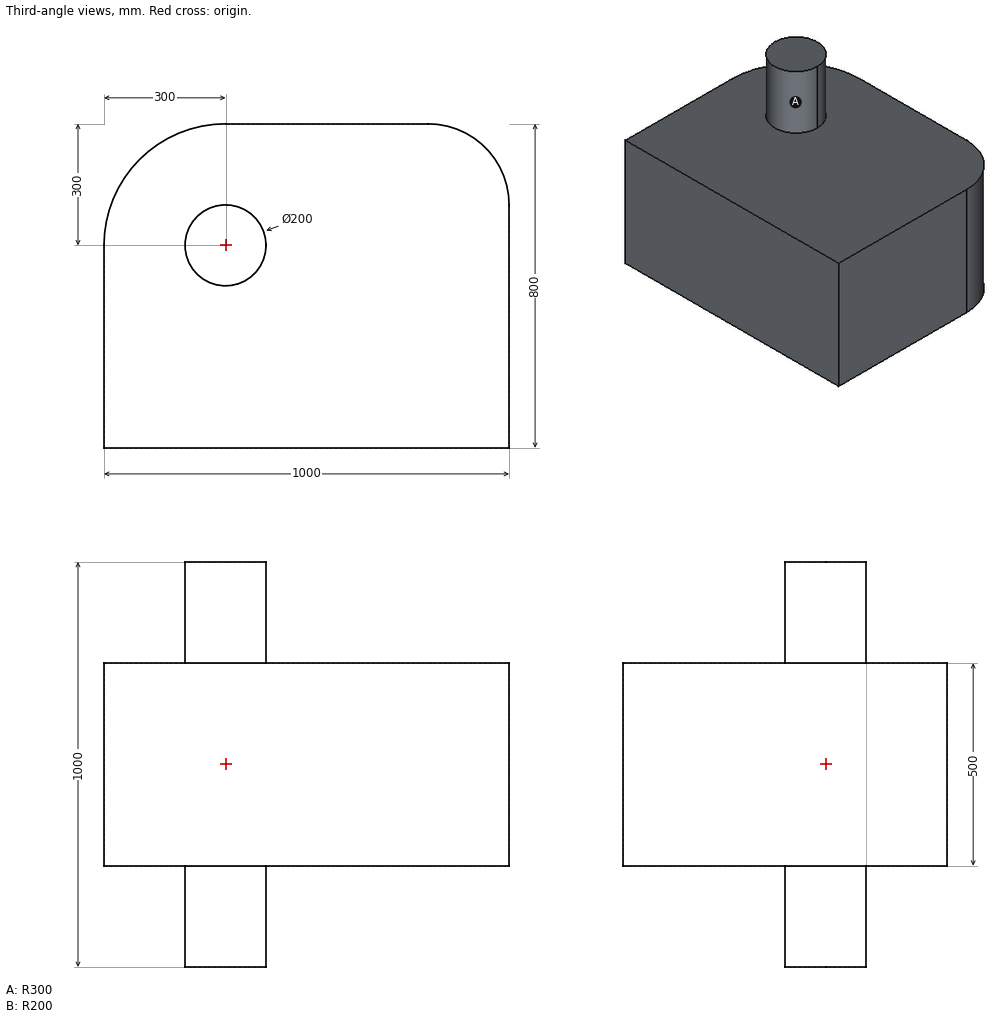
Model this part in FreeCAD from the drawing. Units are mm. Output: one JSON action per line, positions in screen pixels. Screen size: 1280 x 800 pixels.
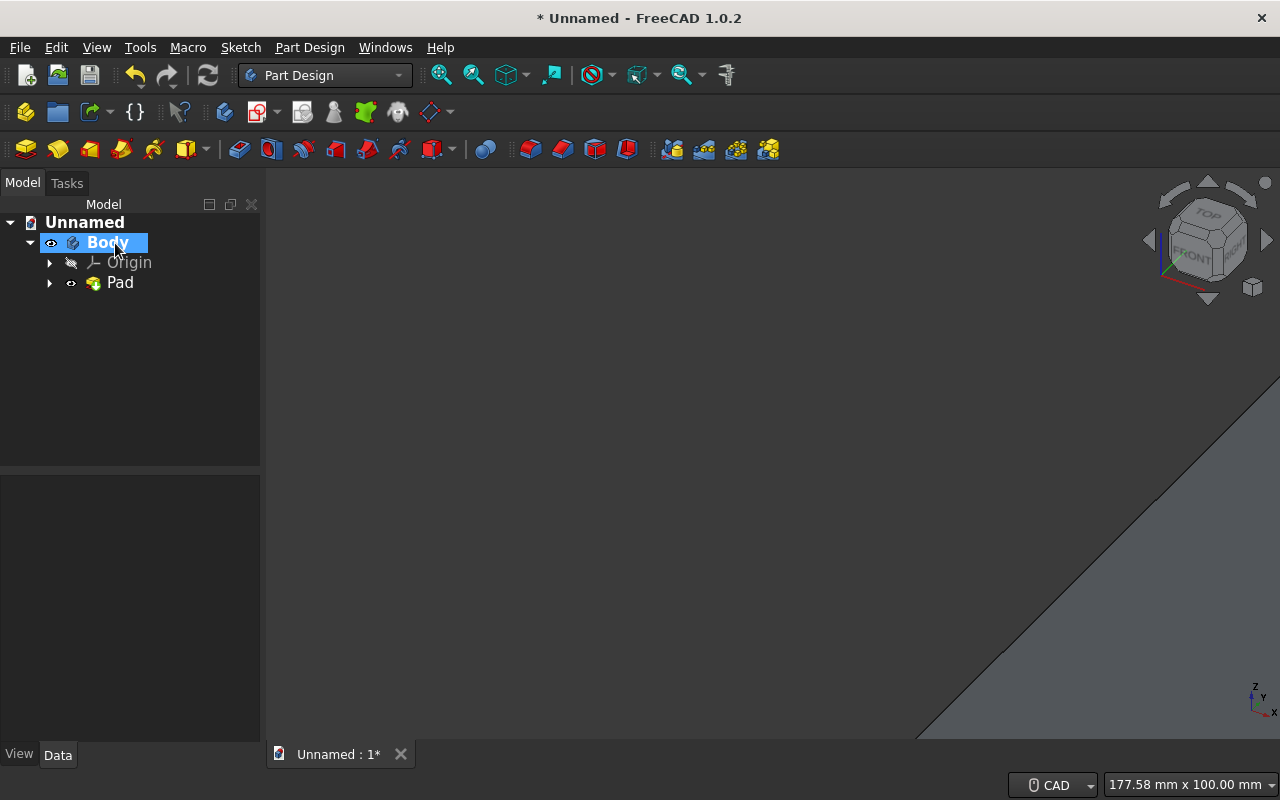
{"action": "left_click", "coordinate": [442, 76]}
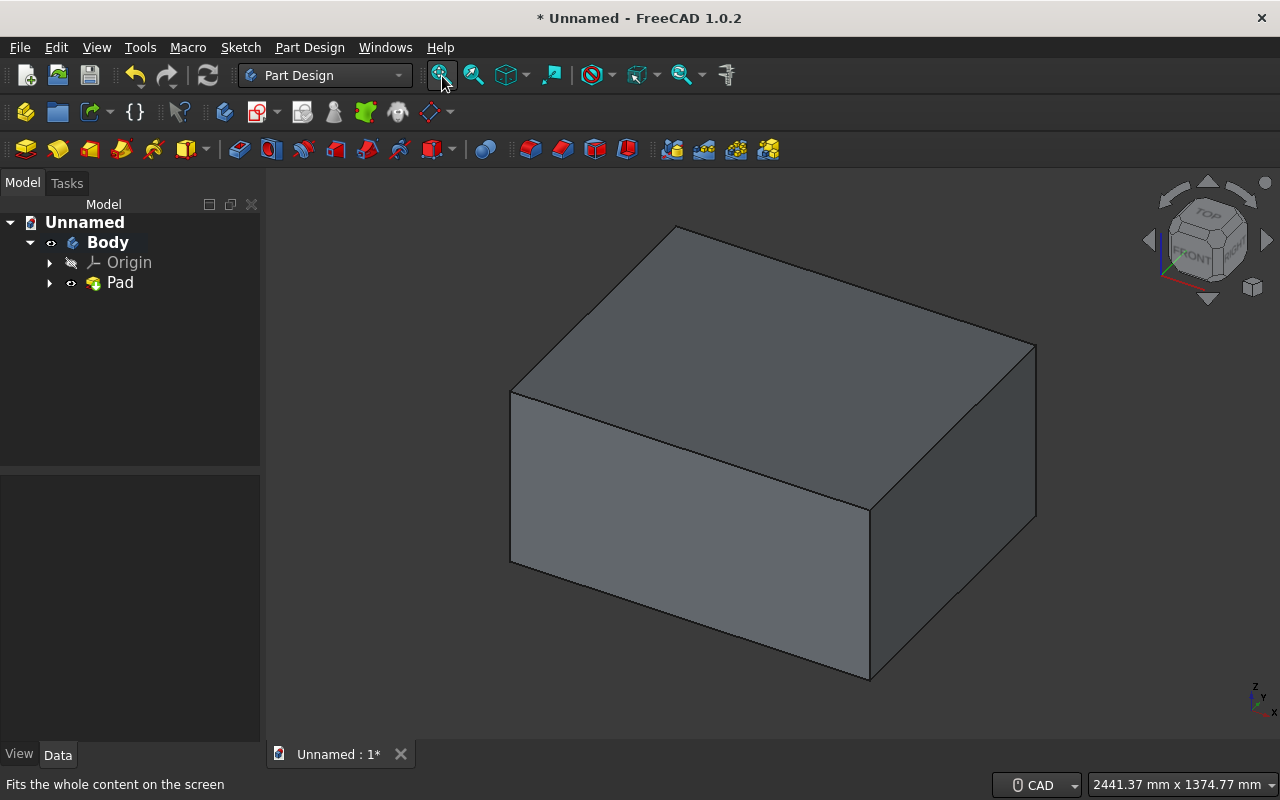
{"action": "left_click", "coordinate": [258, 112]}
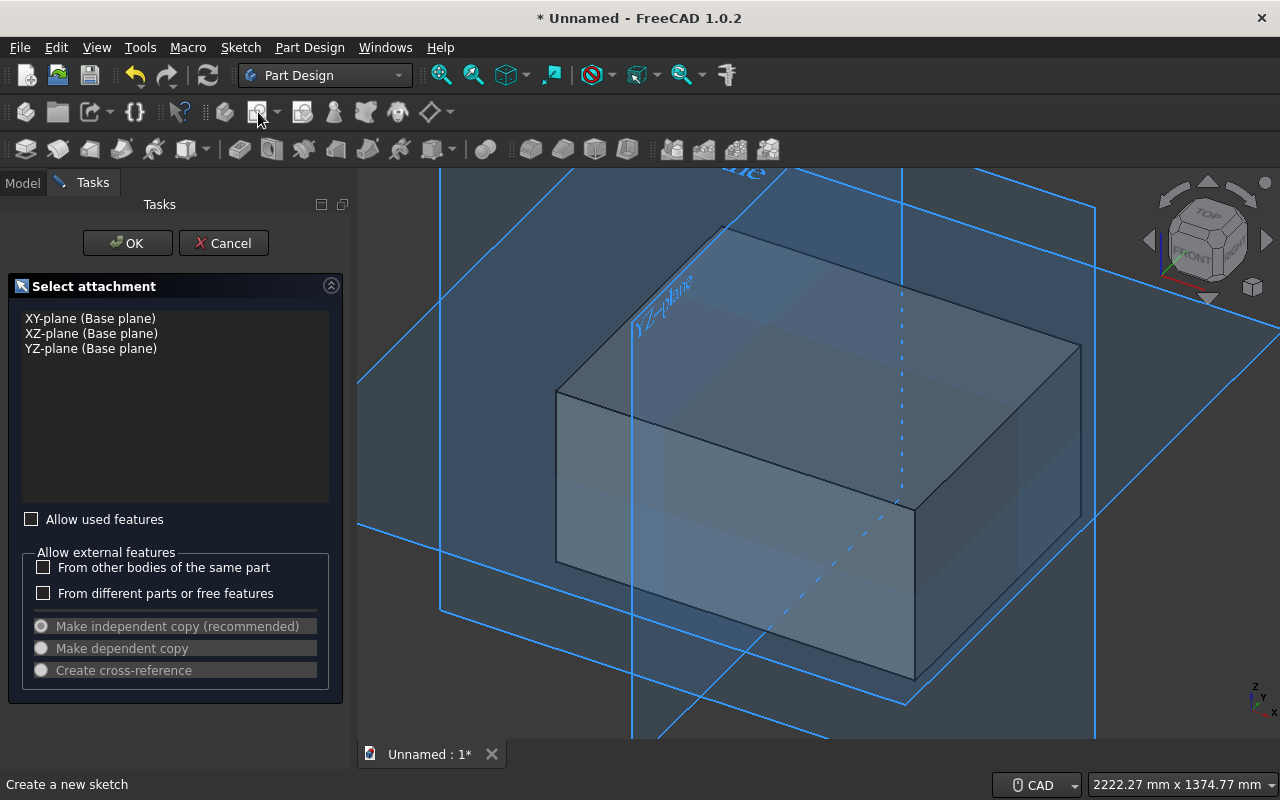
{"action": "left_click", "coordinate": [82, 318]}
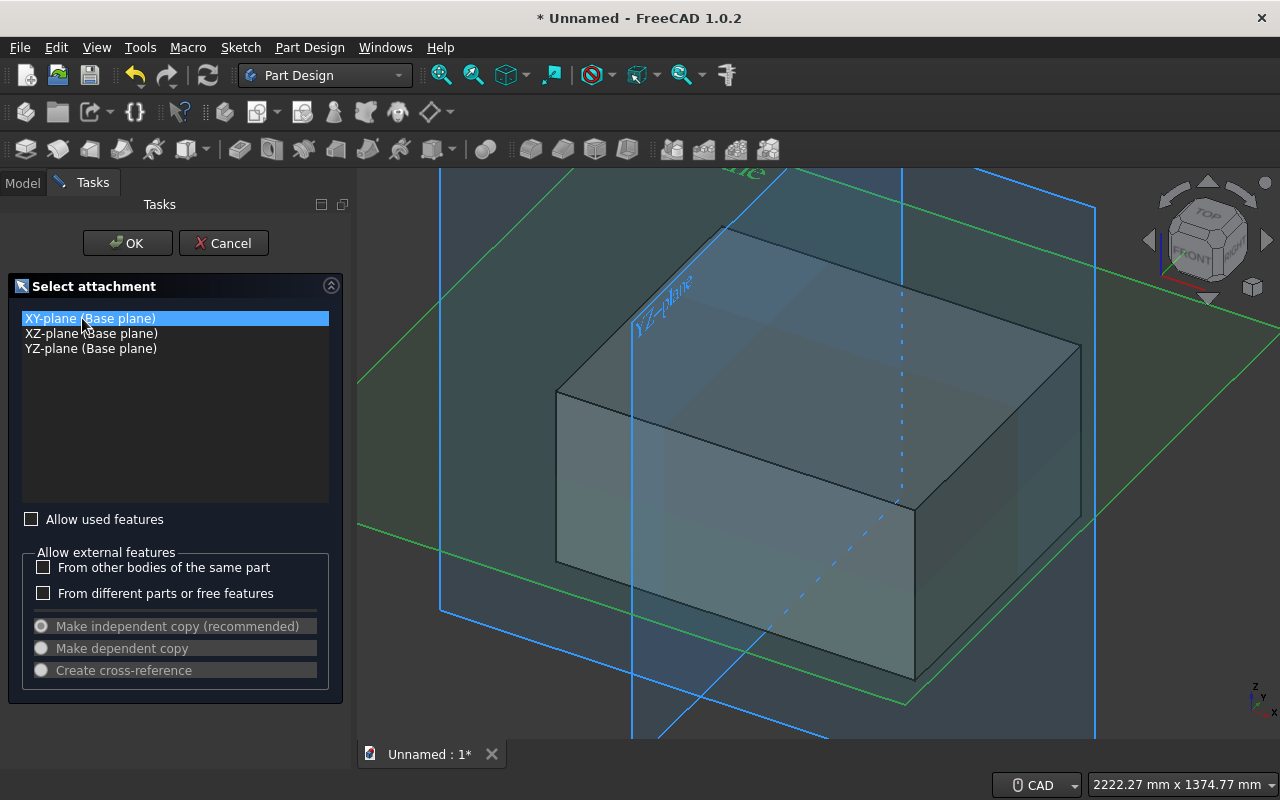
{"action": "left_click", "coordinate": [128, 243]}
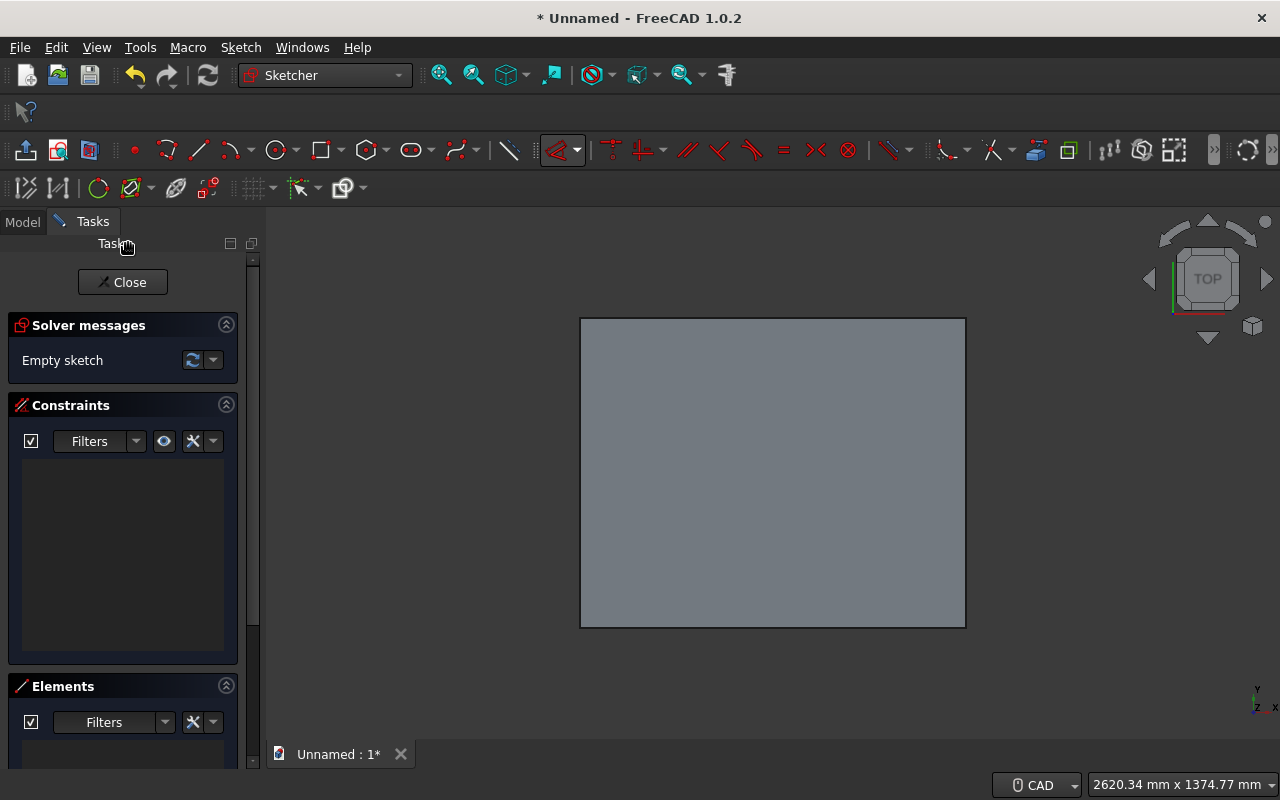
{"action": "left_click", "coordinate": [90, 150]}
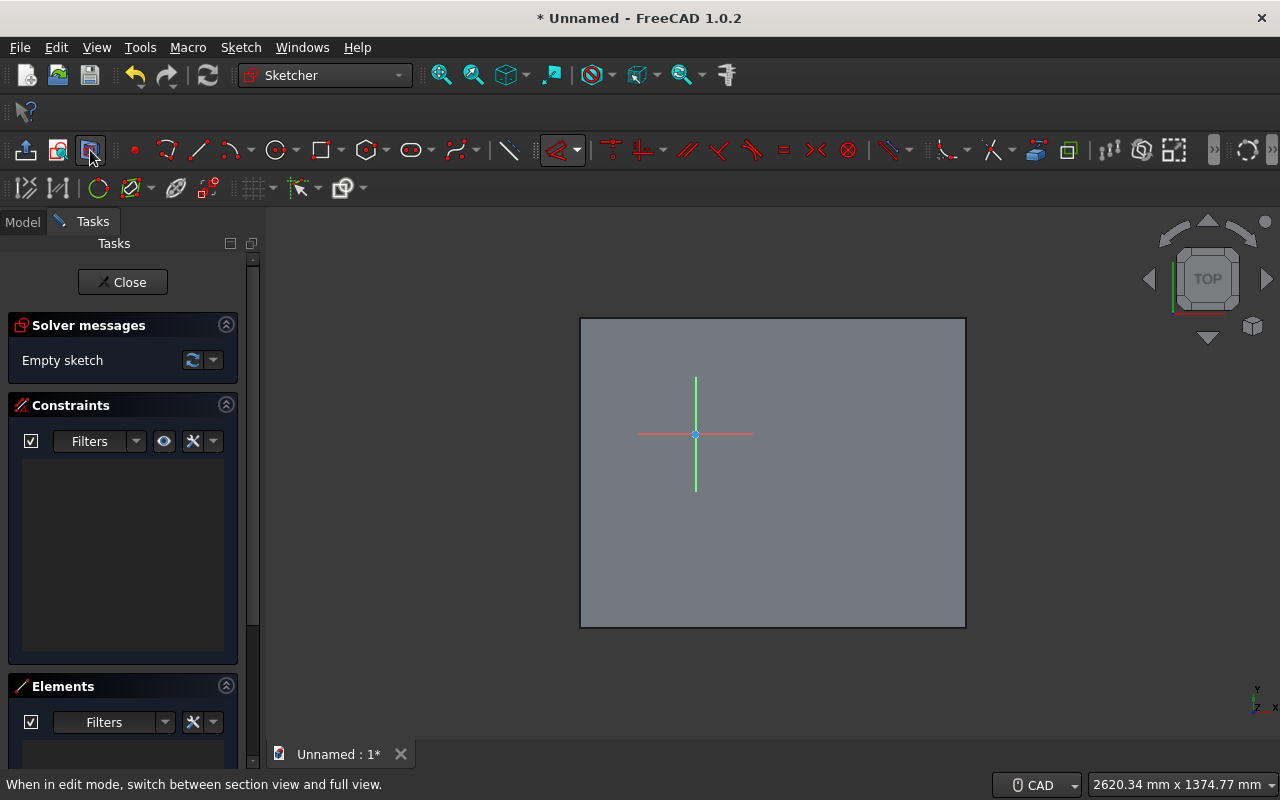
{"action": "scroll", "coordinate": [693, 422], "scroll_direction": "up", "scroll_amount": 7}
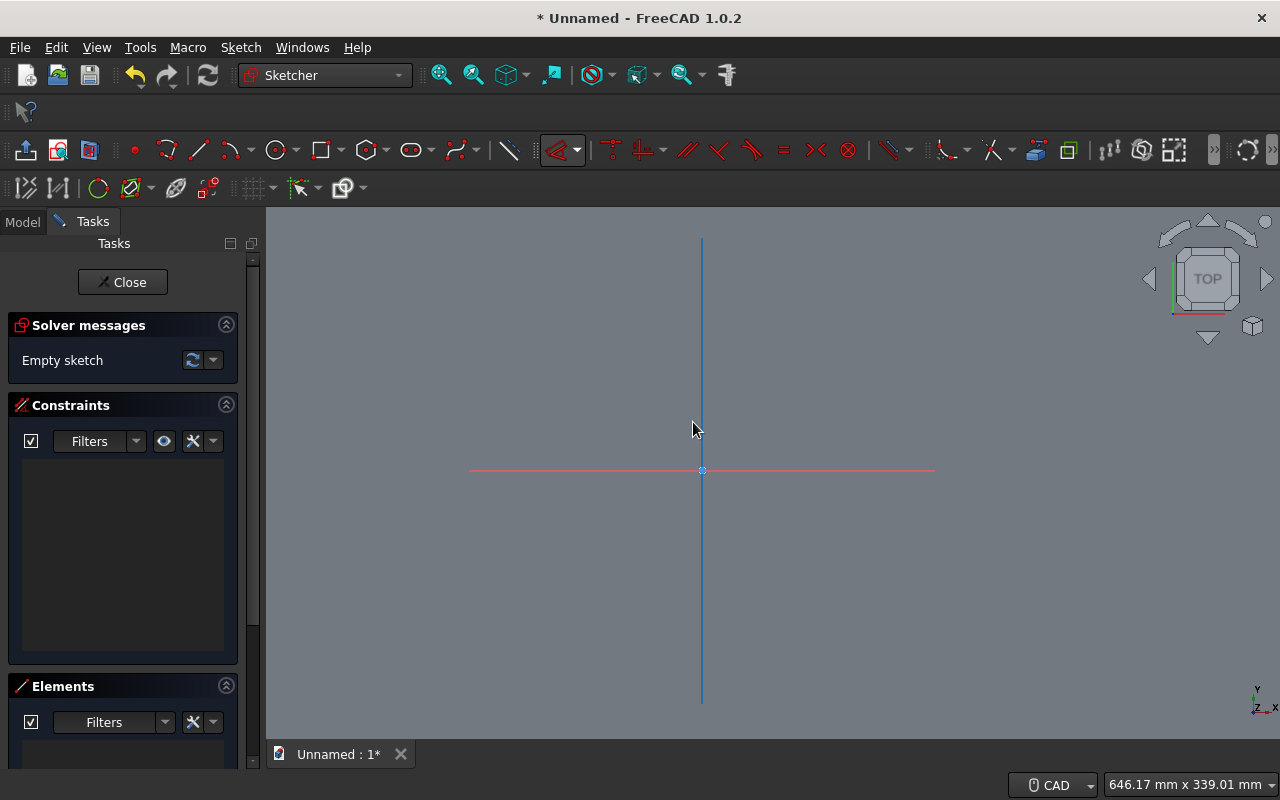
{"action": "key", "text": "g c"}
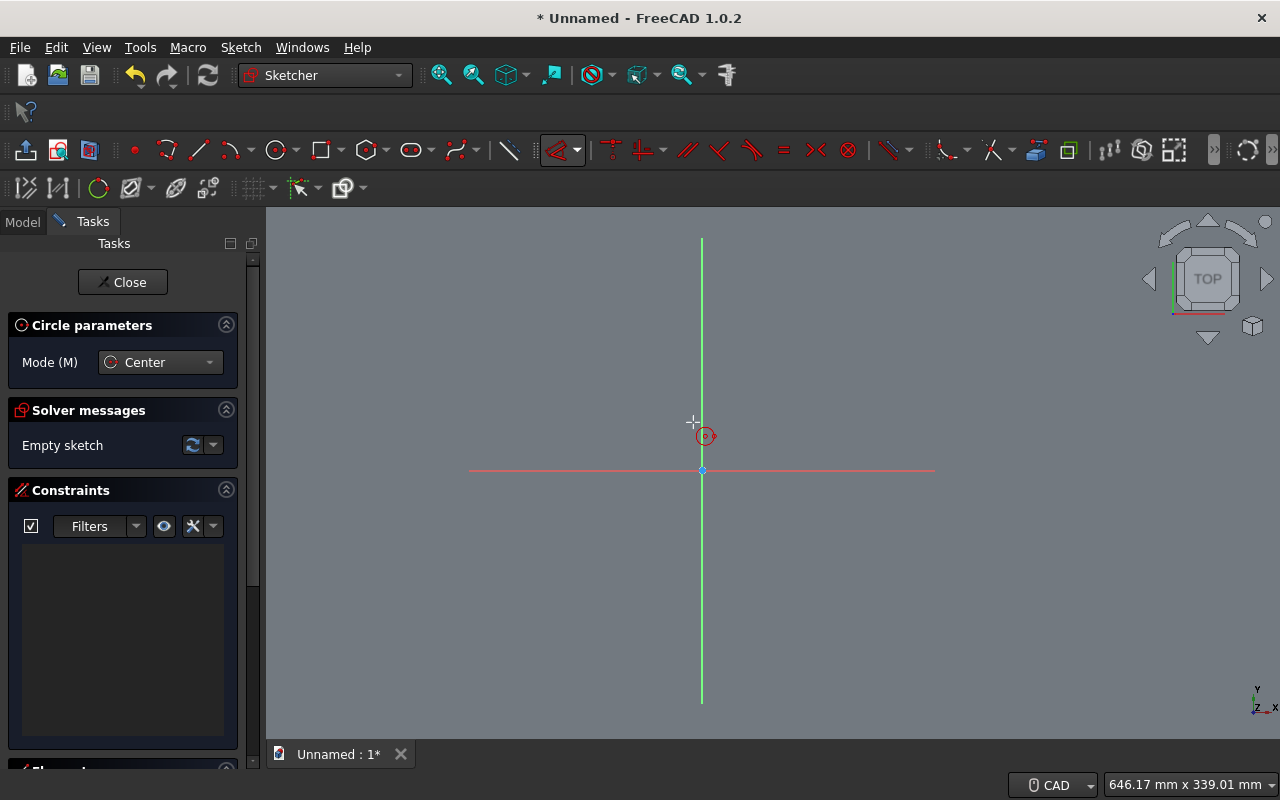
{"action": "left_click", "coordinate": [702, 471]}
{"action": "mouse_move", "coordinate": [813, 360]}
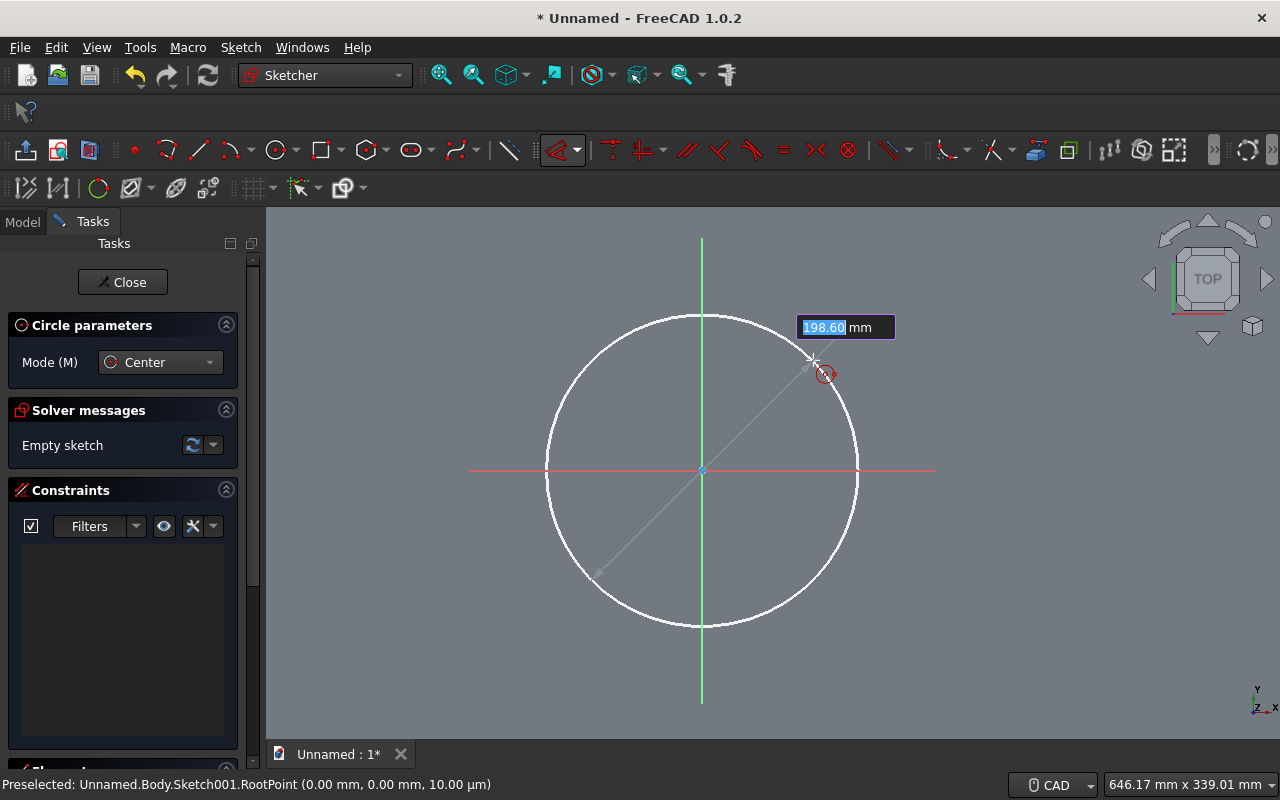
{"action": "type", "text": "200"}
{"action": "key", "text": "Return"}
{"action": "key", "text": "Escape"}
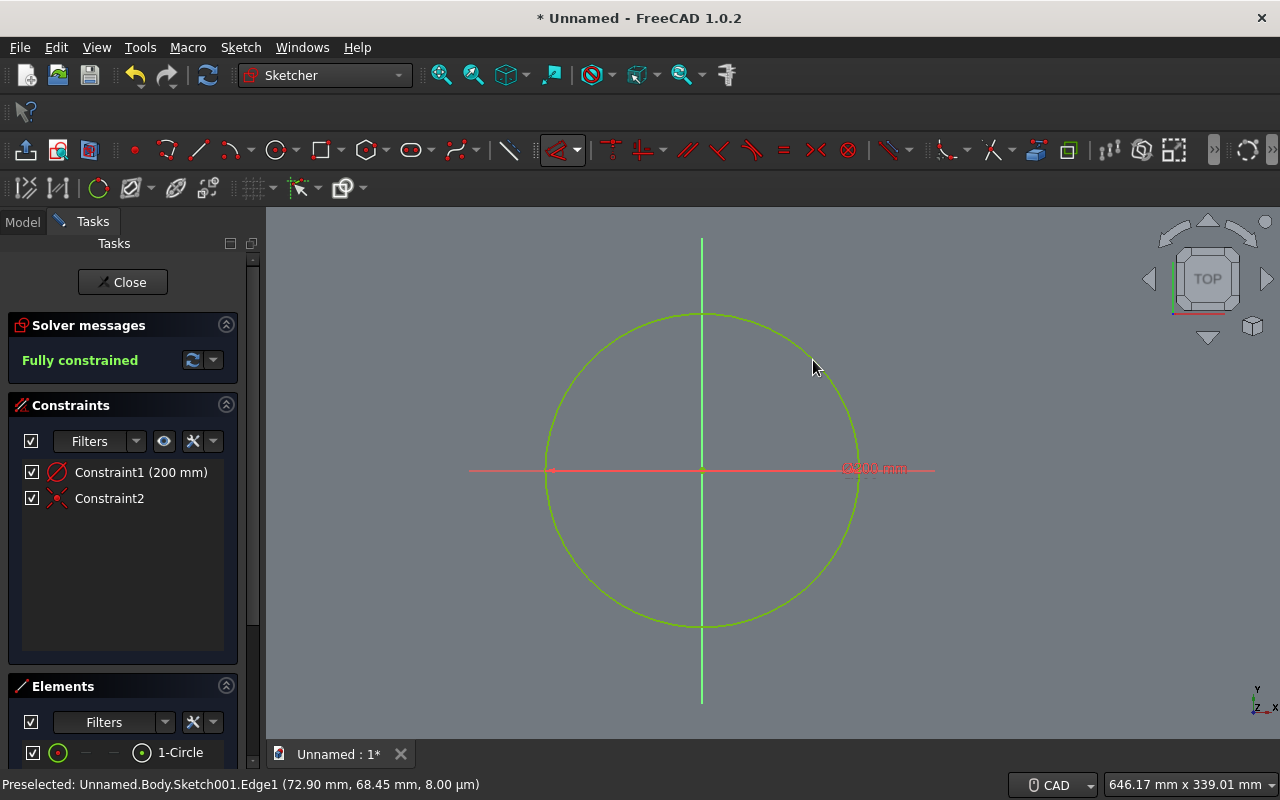
{"action": "left_click", "coordinate": [123, 282]}